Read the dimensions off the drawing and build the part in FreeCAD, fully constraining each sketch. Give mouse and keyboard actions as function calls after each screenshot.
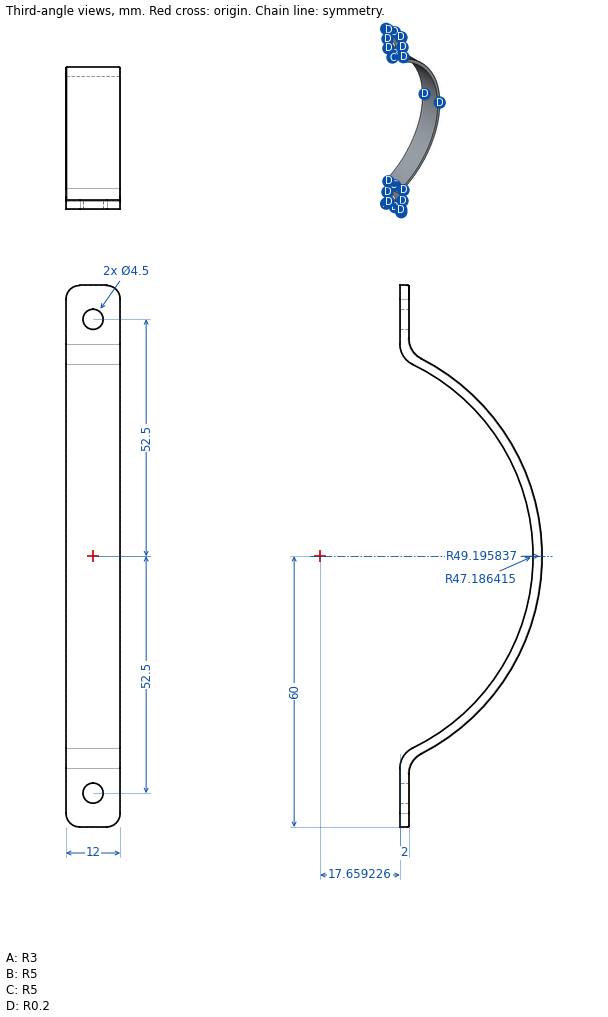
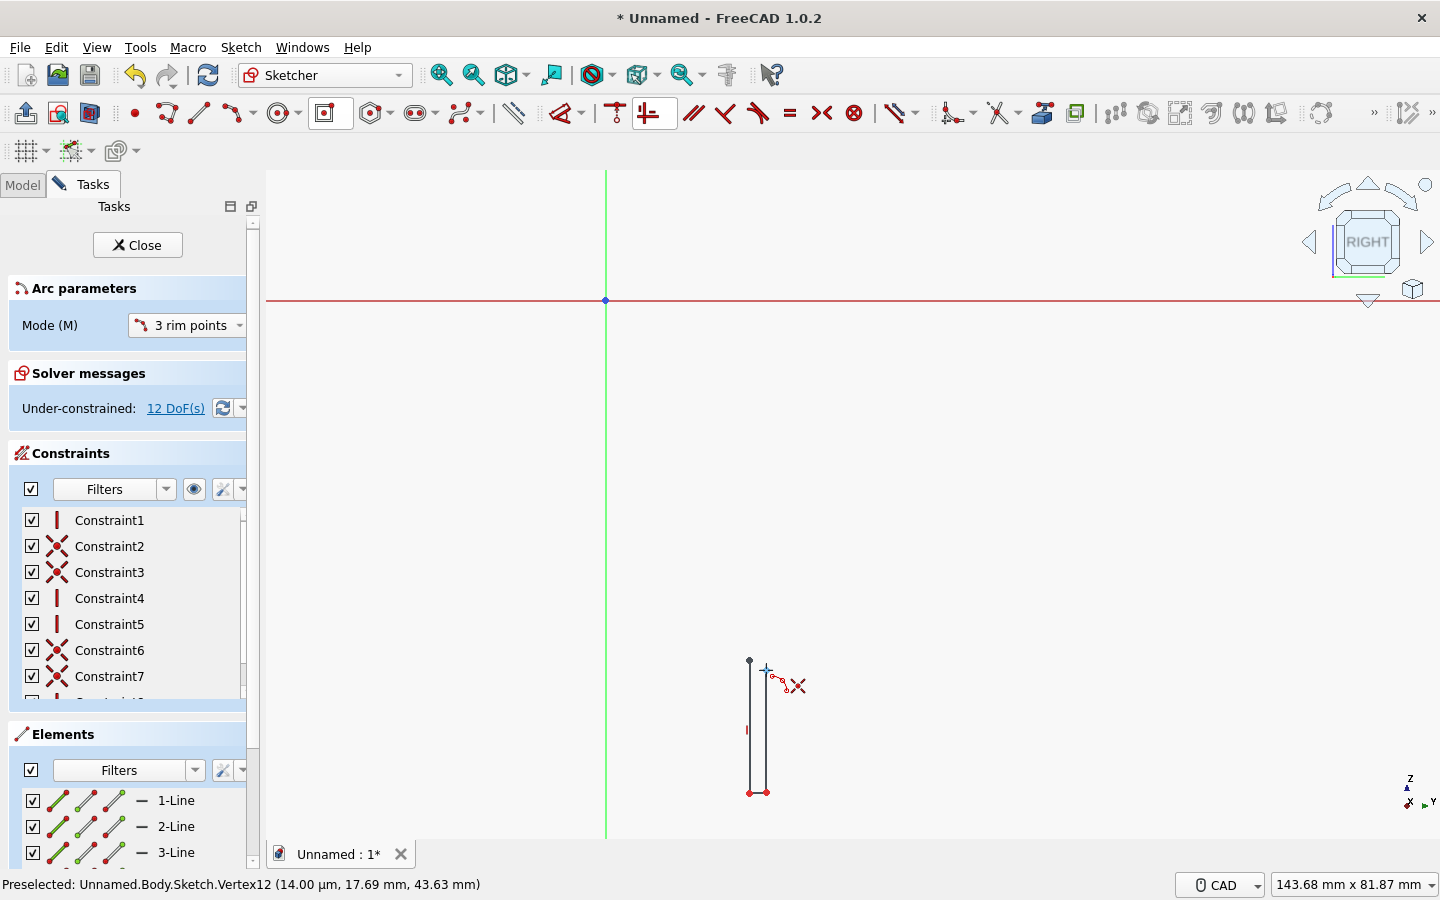
click(766, 671)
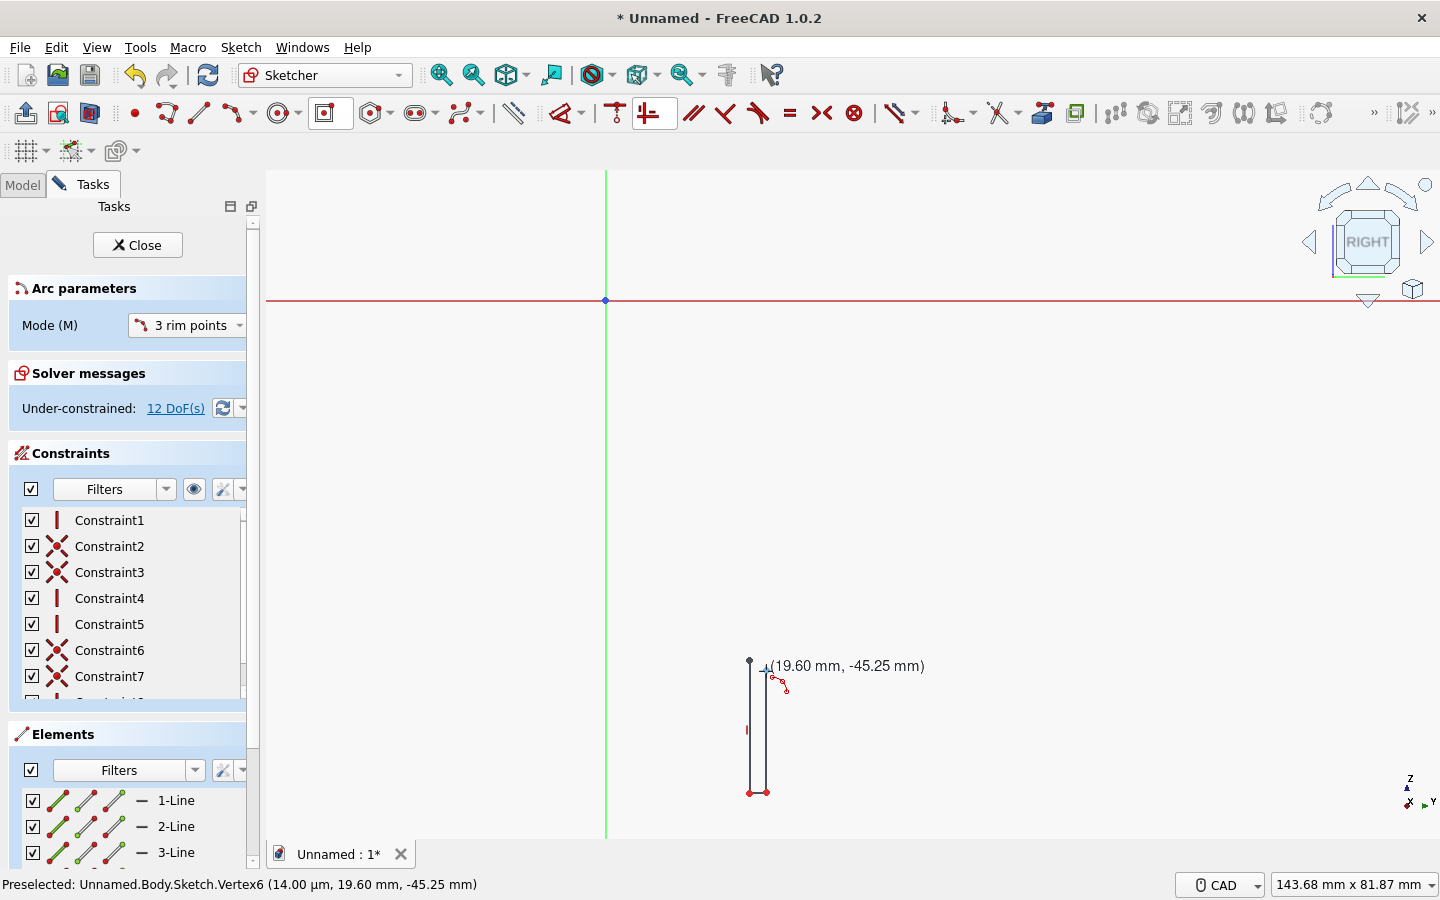
scroll(766, 671, down, 4)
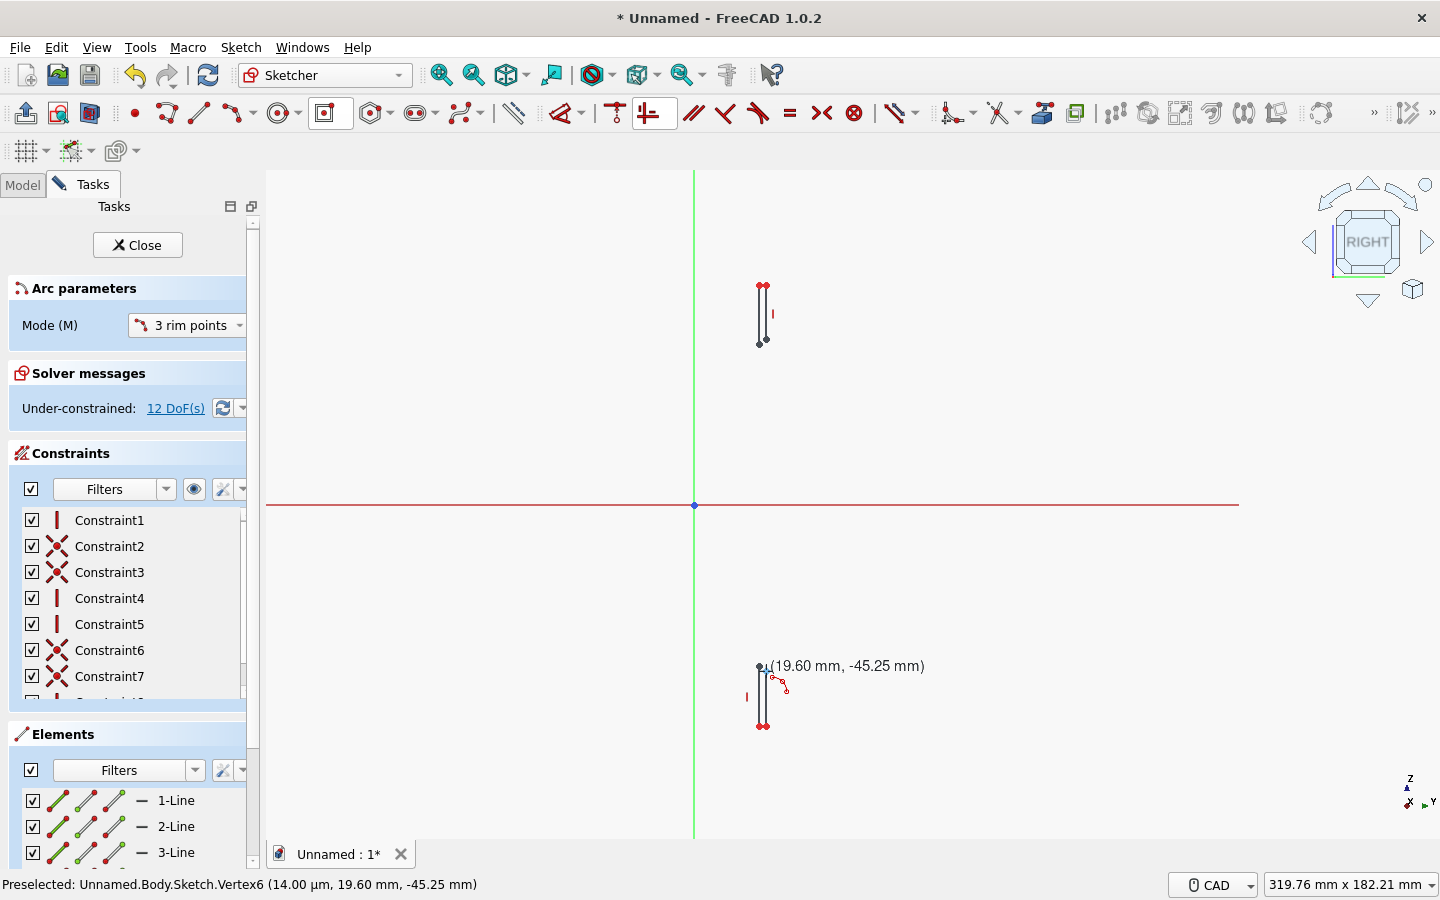
scroll(766, 339, up, 4)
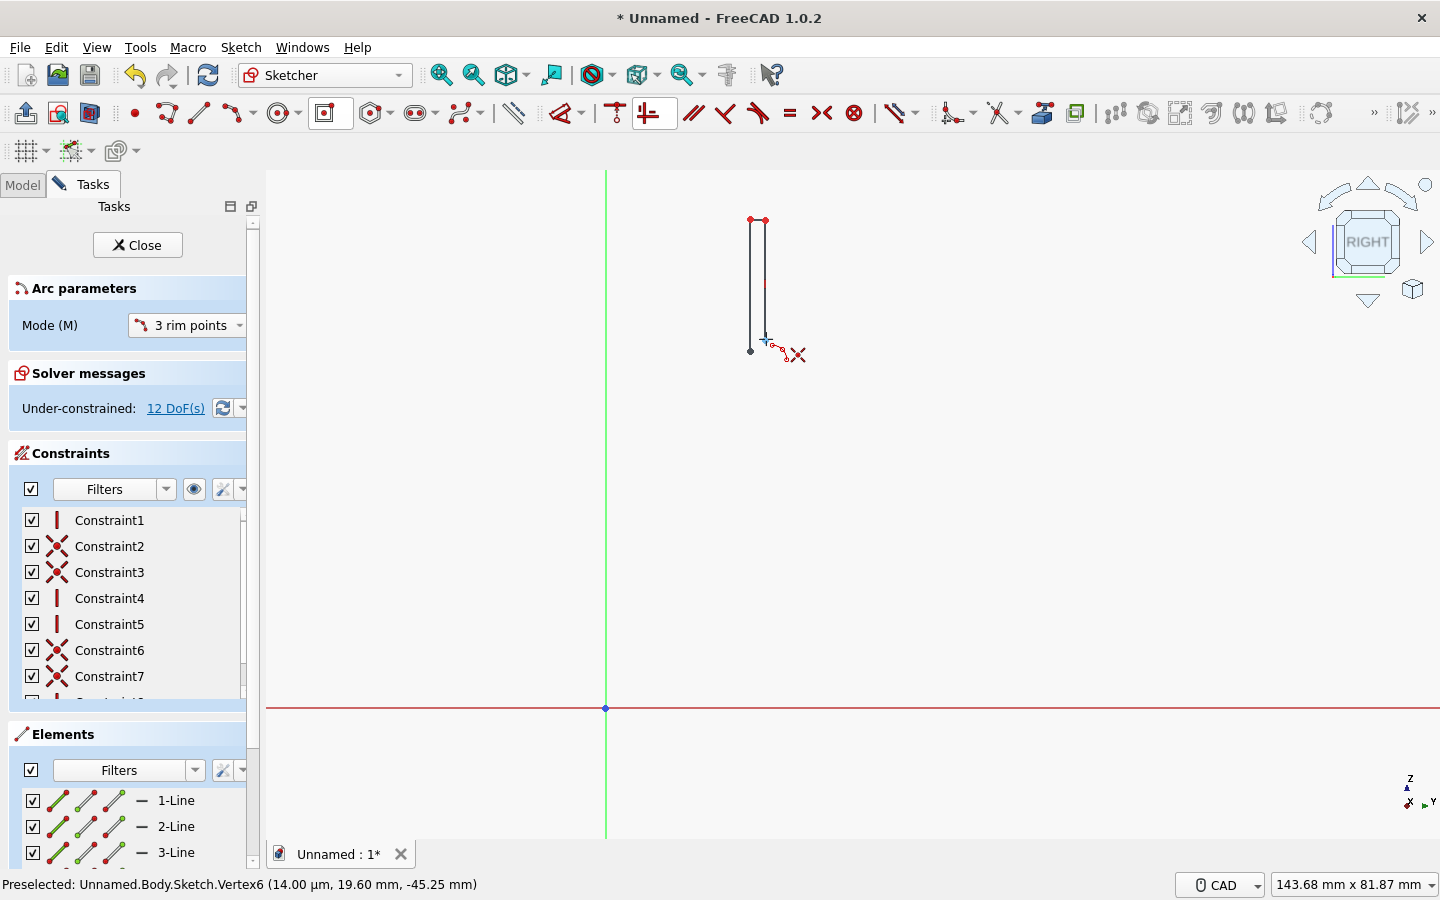
click(765, 341)
click(997, 801)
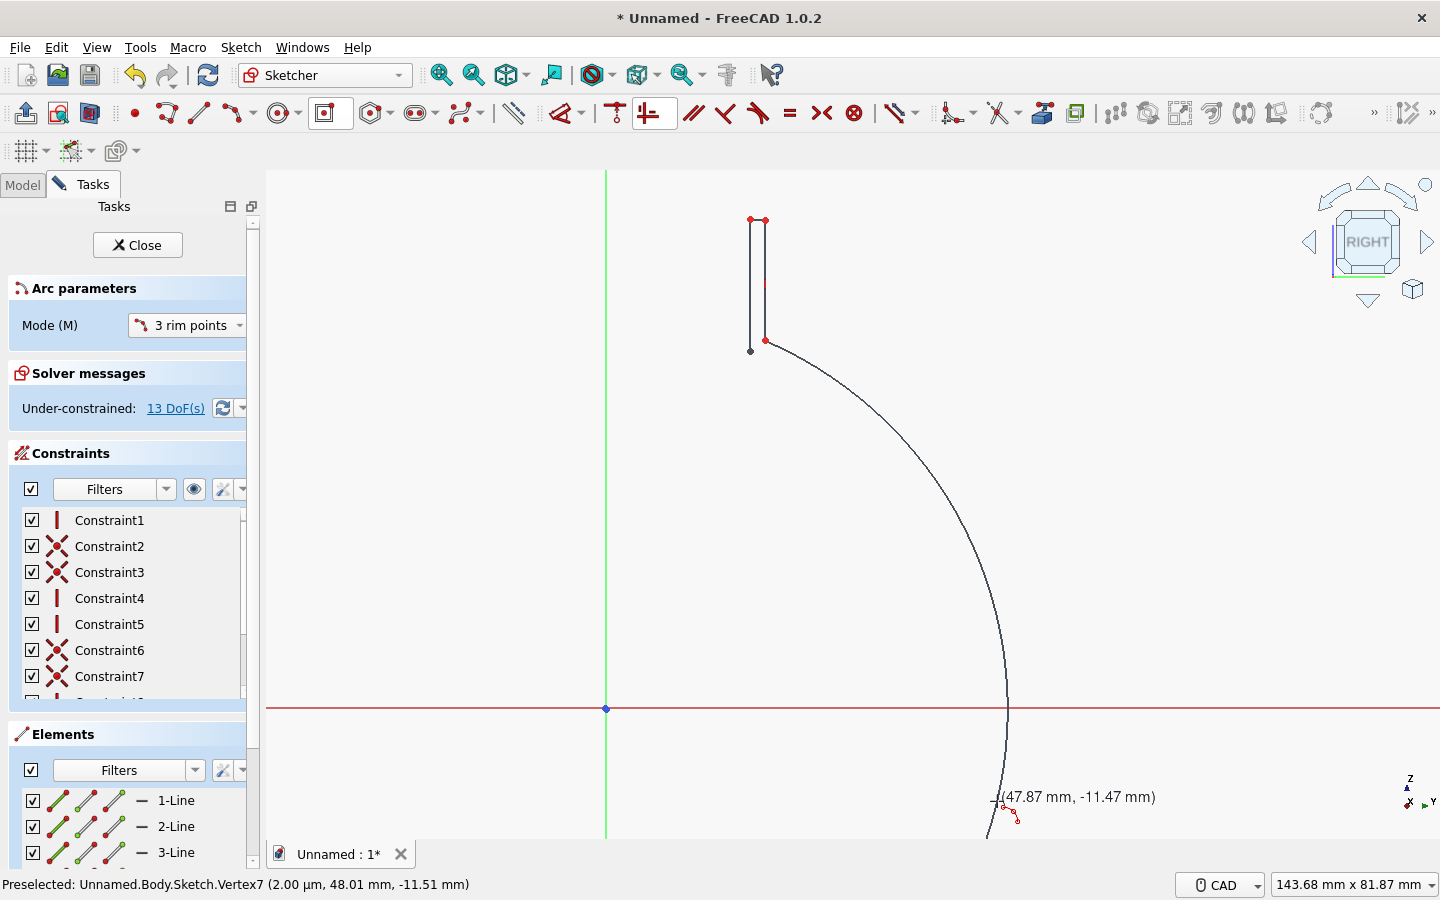
click(750, 352)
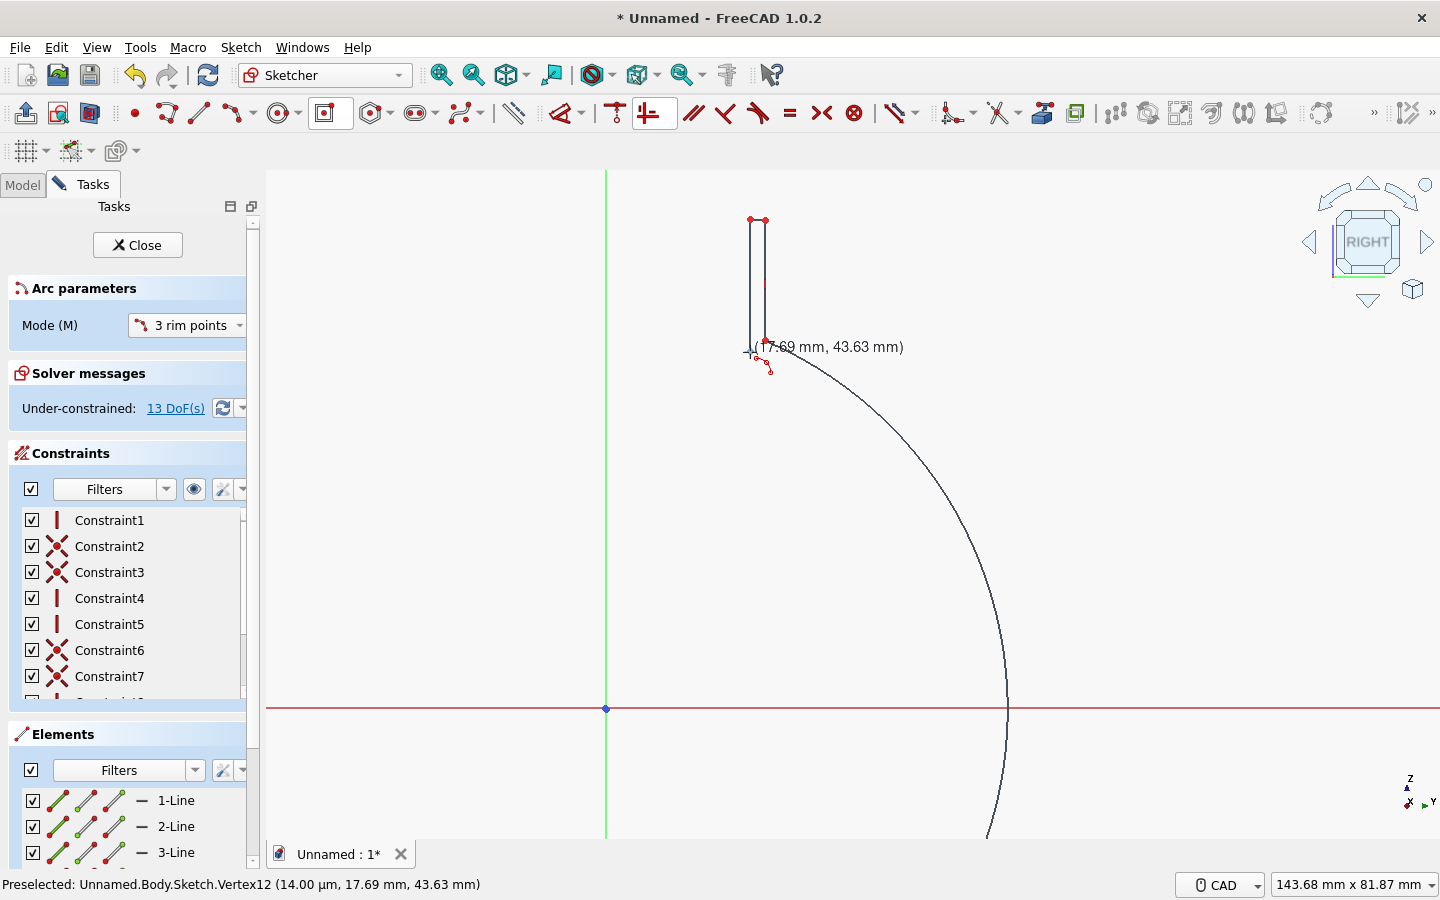
scroll(766, 338, down, 4)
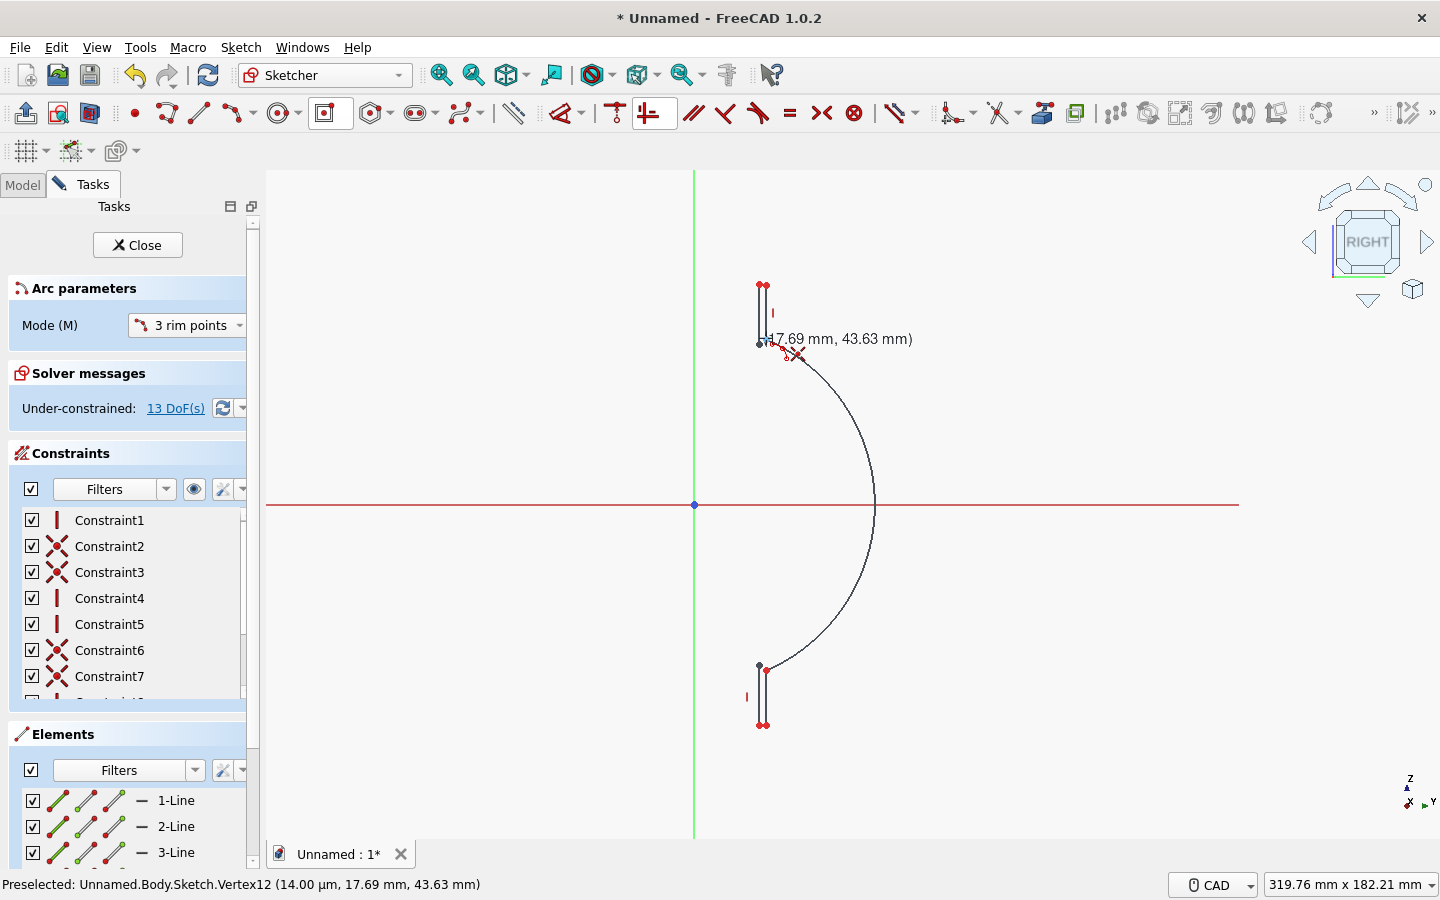
scroll(759, 665, up, 3)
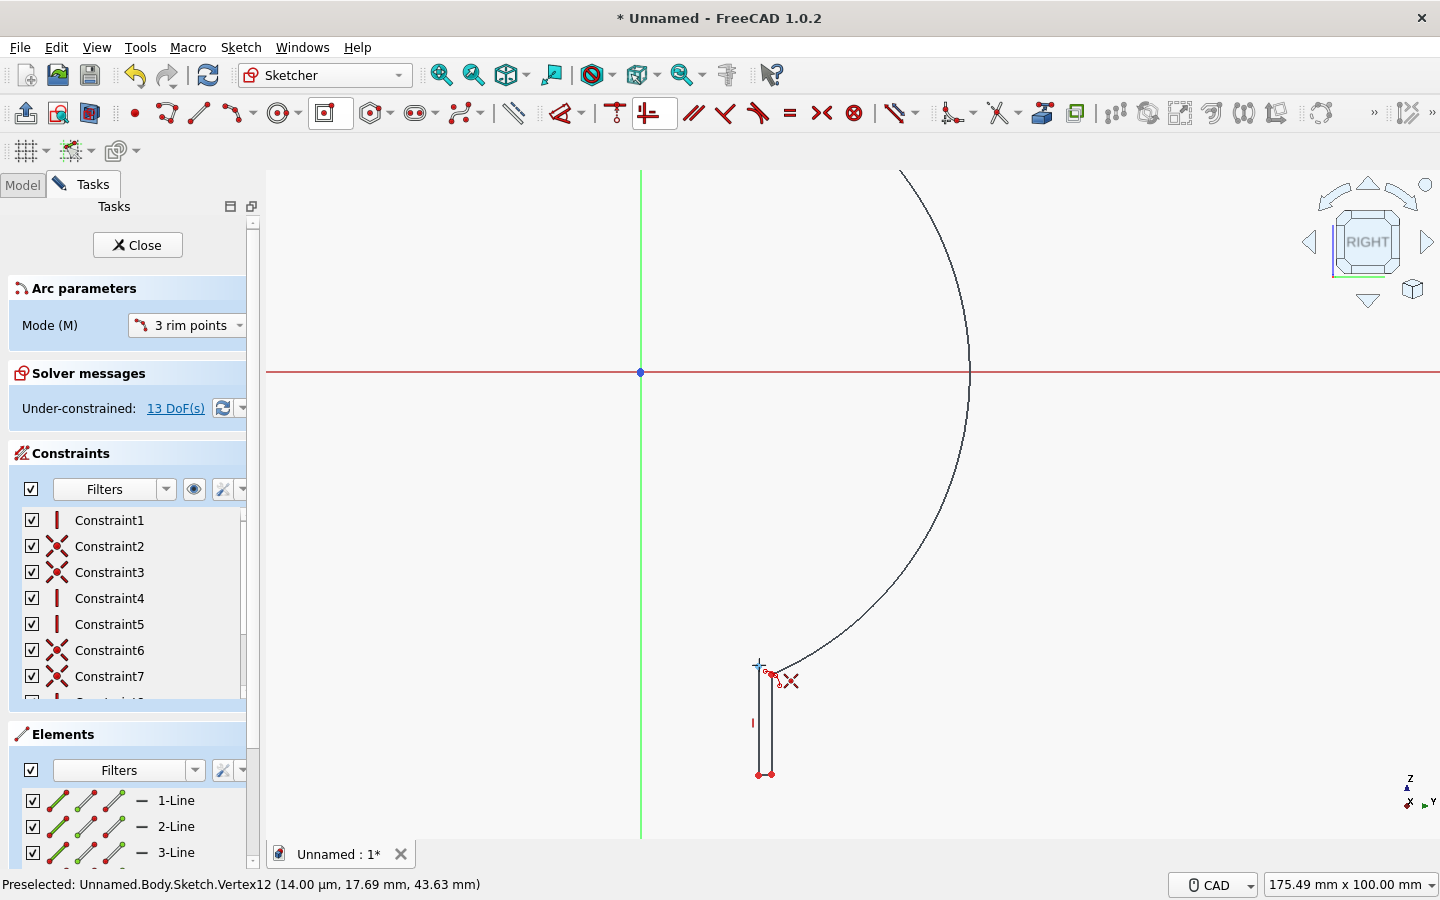
click(759, 666)
click(921, 516)
key(Escape)